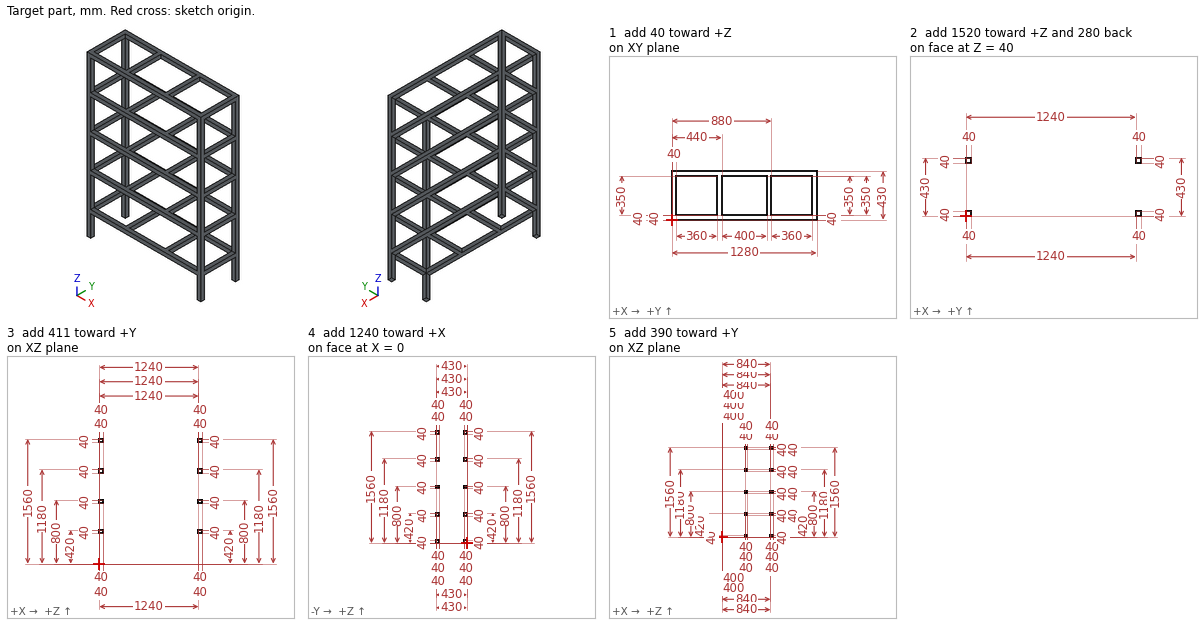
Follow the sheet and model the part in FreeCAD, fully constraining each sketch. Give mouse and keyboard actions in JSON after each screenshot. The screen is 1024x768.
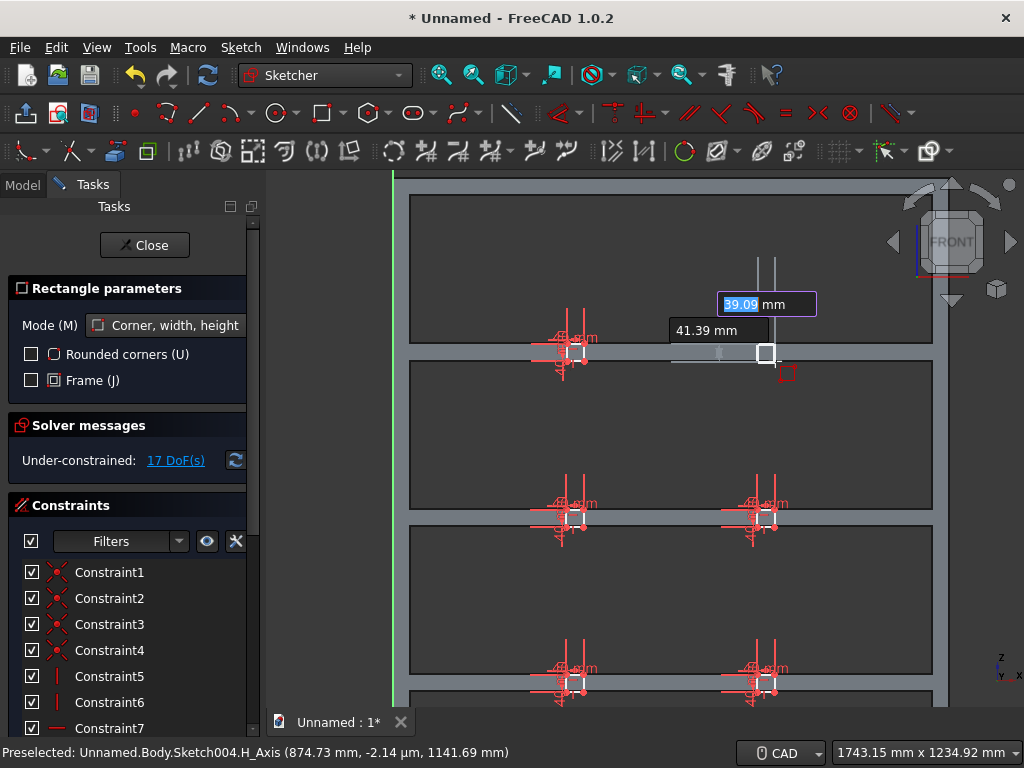
{"action": "type", "text": "40"}
{"action": "key", "text": "Tab"}
{"action": "type", "text": "40"}
{"action": "key", "text": "Return"}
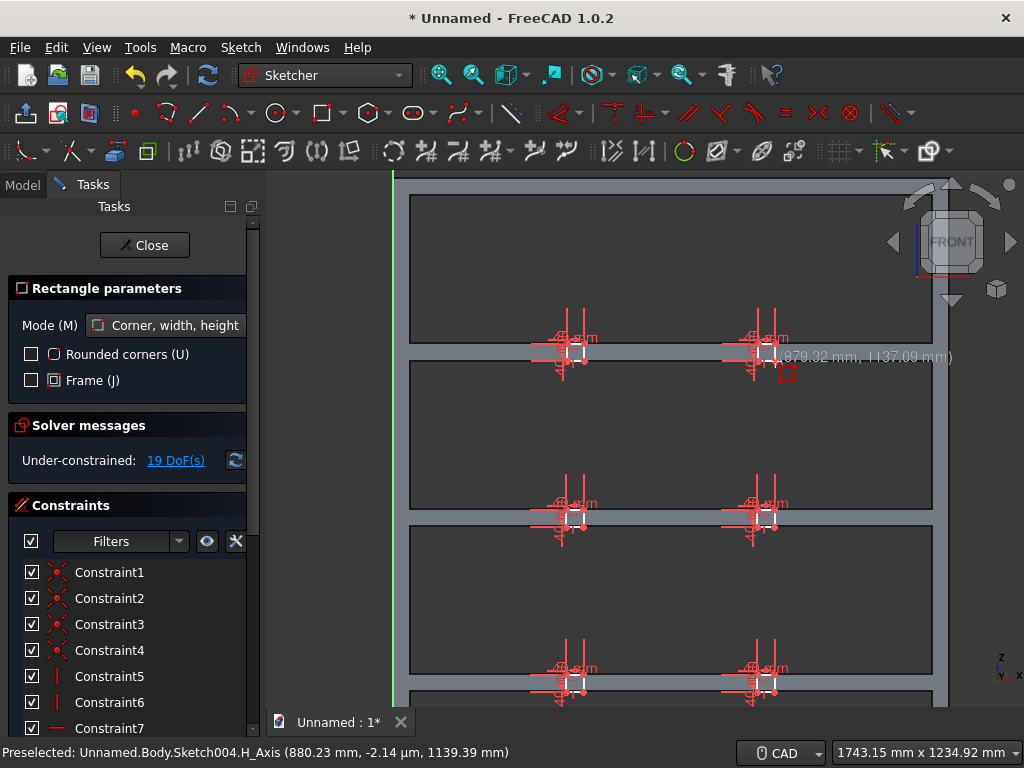
{"action": "scroll", "coordinate": [567, 343], "scroll_direction": "down", "scroll_amount": 3}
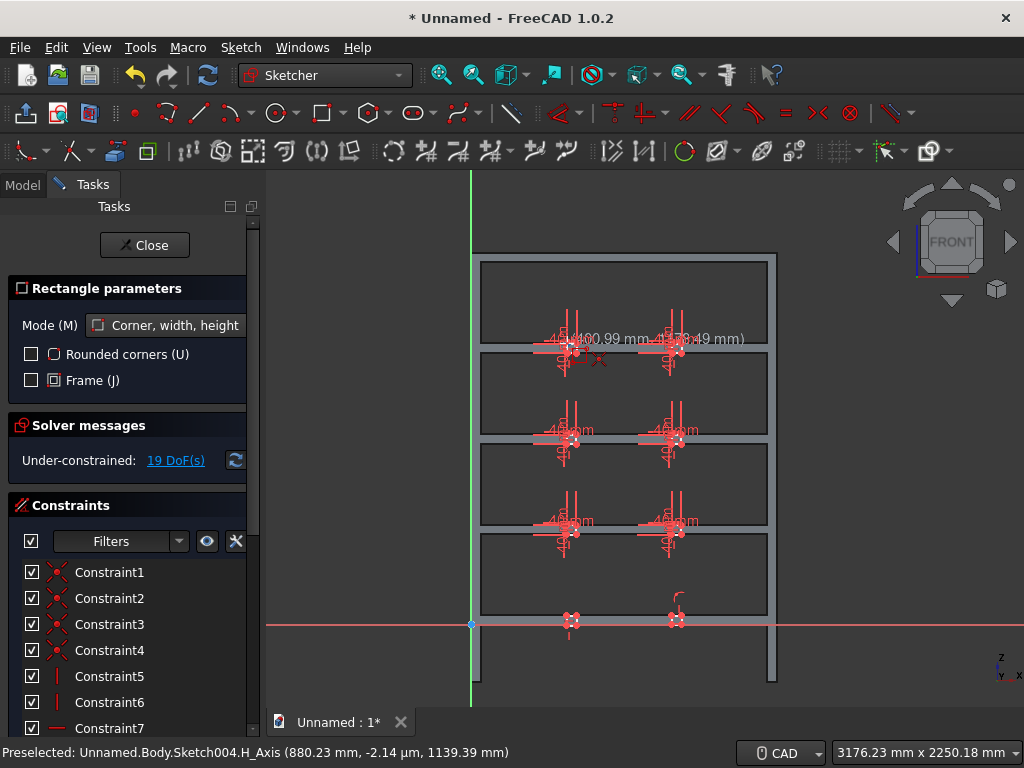
{"action": "scroll", "coordinate": [672, 253], "scroll_direction": "up", "scroll_amount": 3}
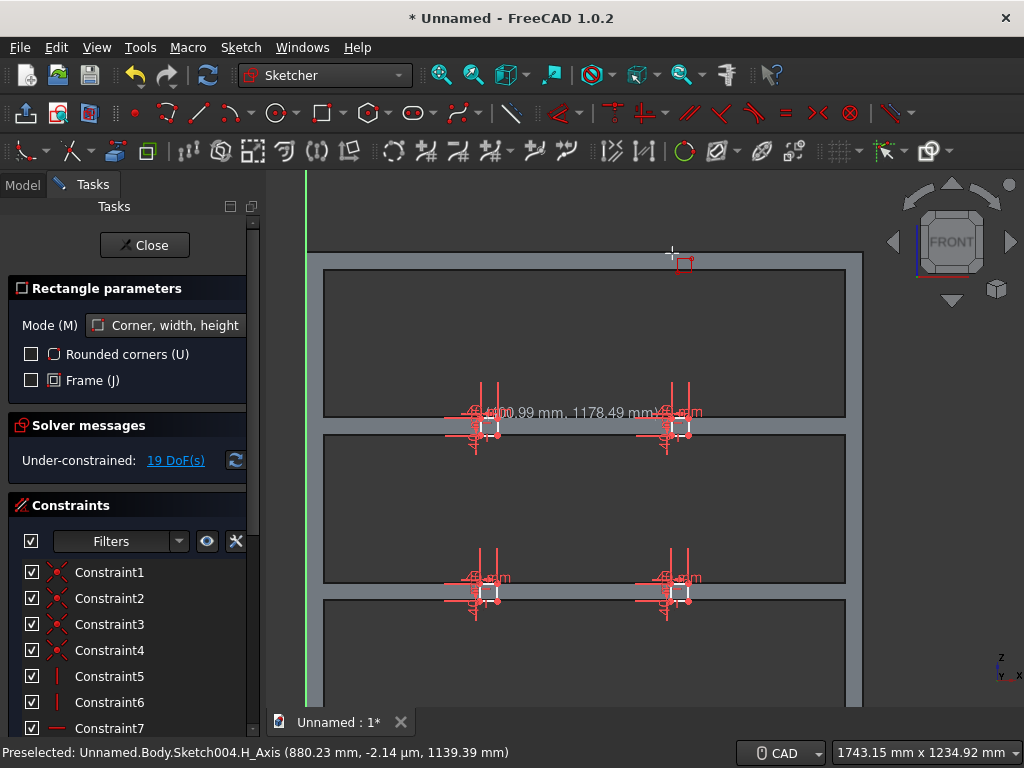
{"action": "left_click", "coordinate": [671, 252]}
{"action": "mouse_move", "coordinate": [689, 270]}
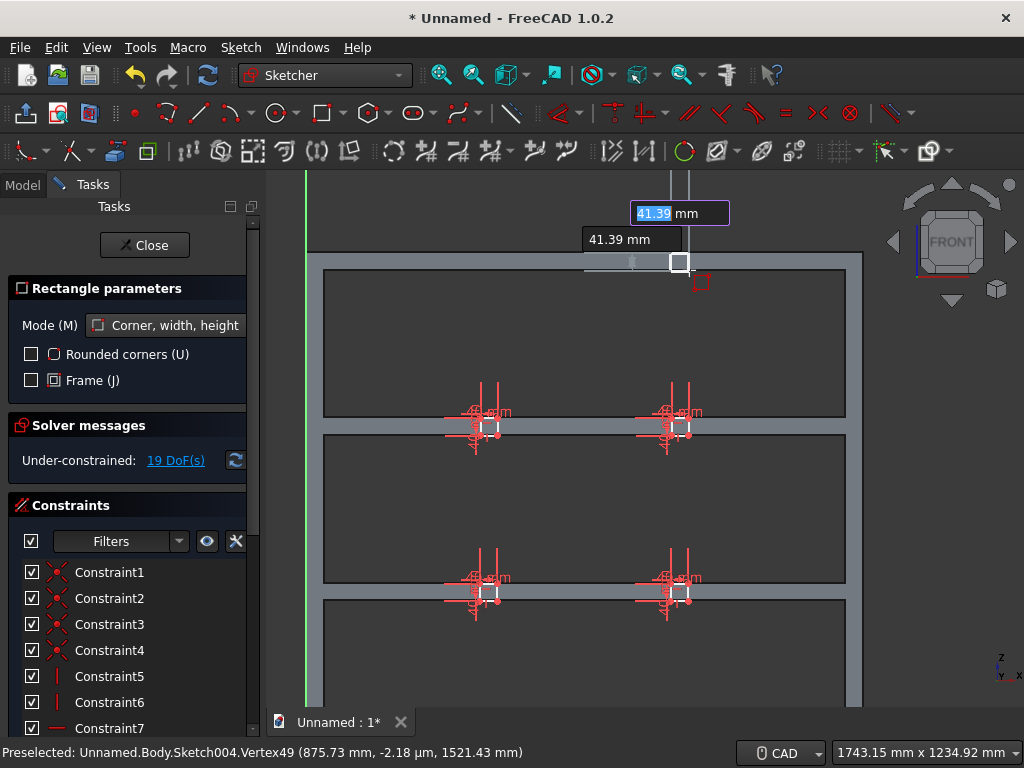
{"action": "type", "text": "40"}
{"action": "key", "text": "Tab"}
{"action": "type", "text": "40"}
{"action": "key", "text": "Return"}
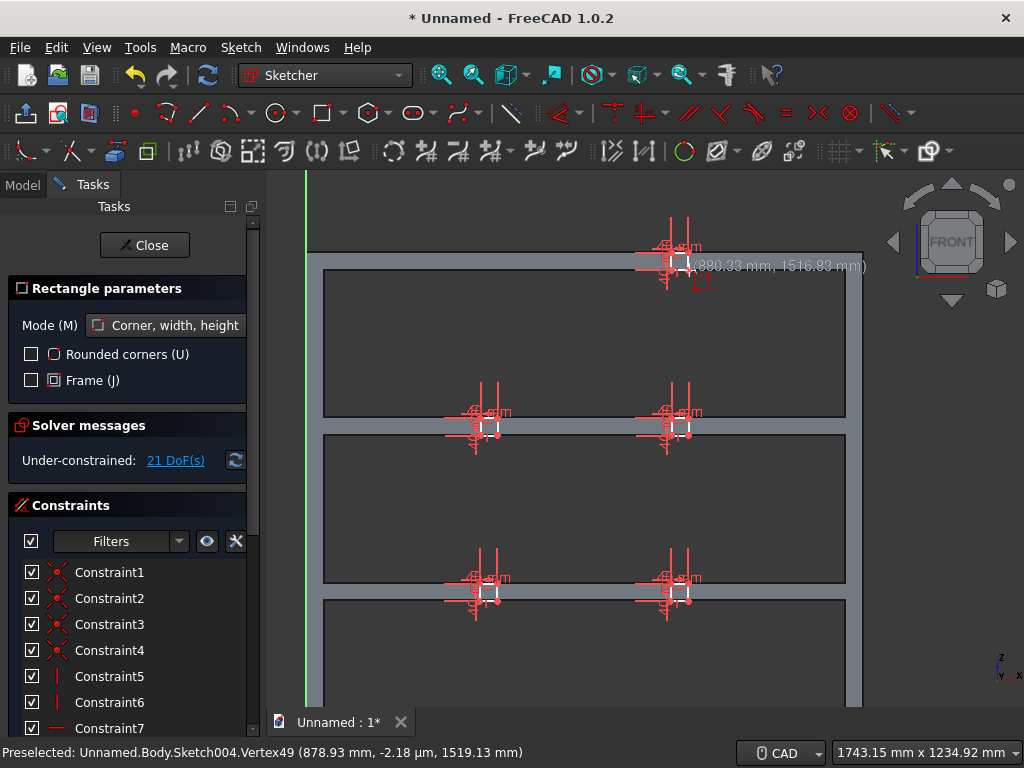
{"action": "left_click", "coordinate": [480, 252]}
{"action": "mouse_move", "coordinate": [498, 270]}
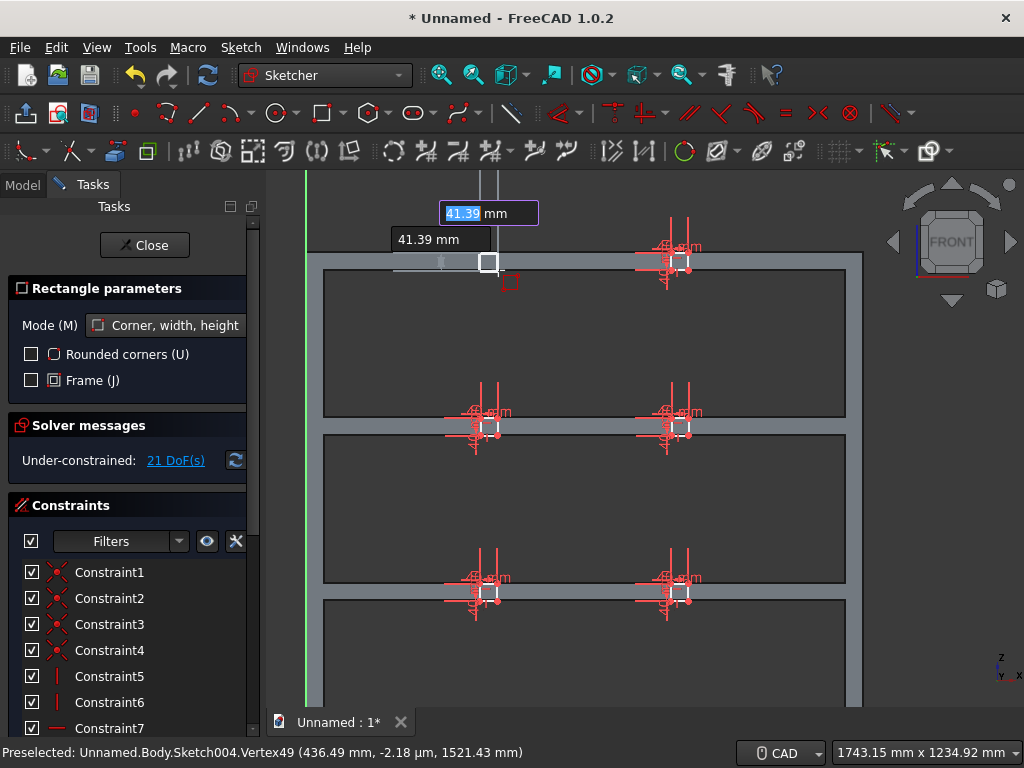
{"action": "type", "text": "40"}
{"action": "key", "text": "Tab"}
{"action": "type", "text": "40"}
{"action": "key", "text": "Return"}
{"action": "key", "text": "Escape"}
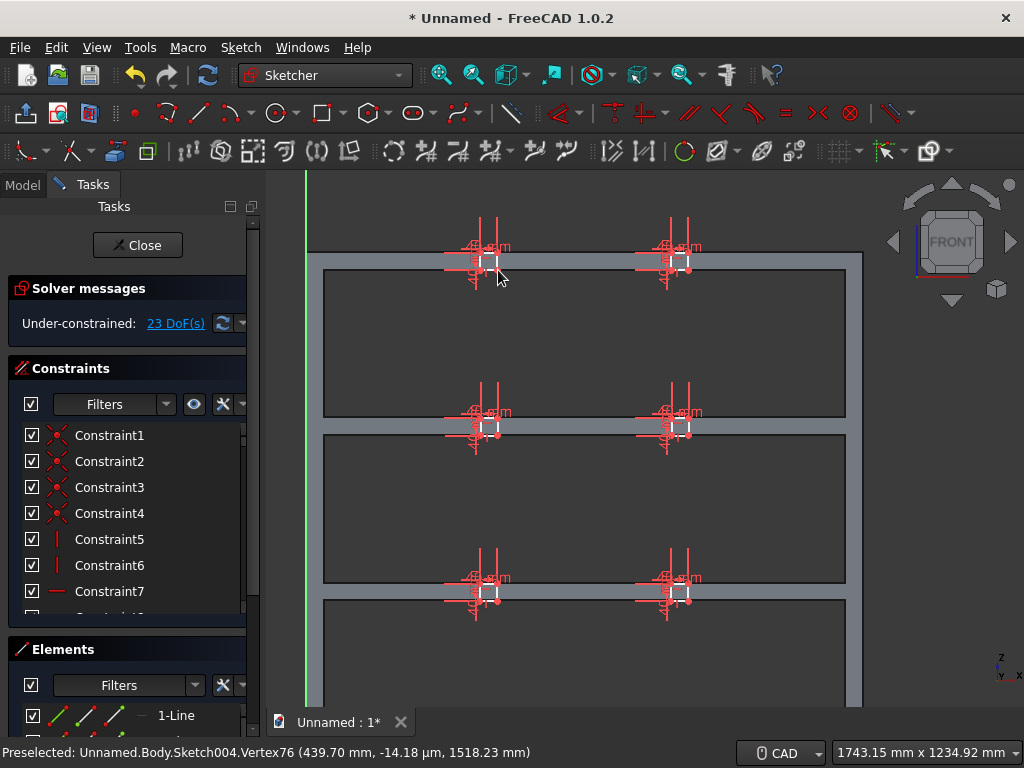
{"action": "scroll", "coordinate": [673, 253], "scroll_direction": "down", "scroll_amount": 3}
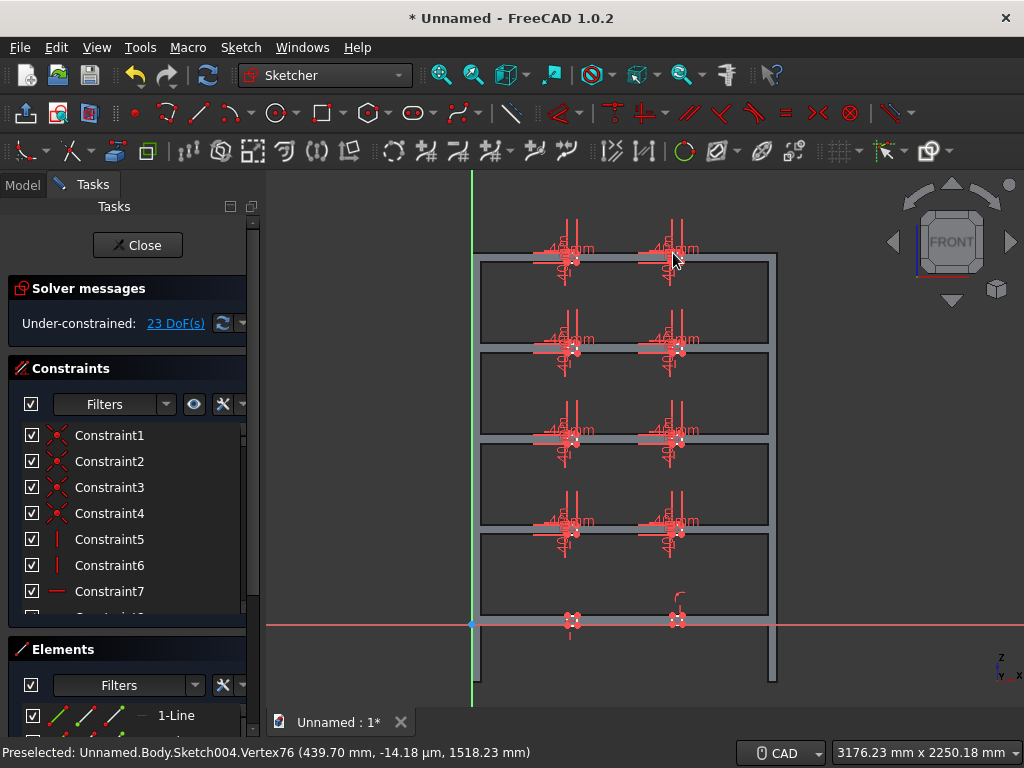
{"action": "scroll", "coordinate": [567, 626], "scroll_direction": "up", "scroll_amount": 2}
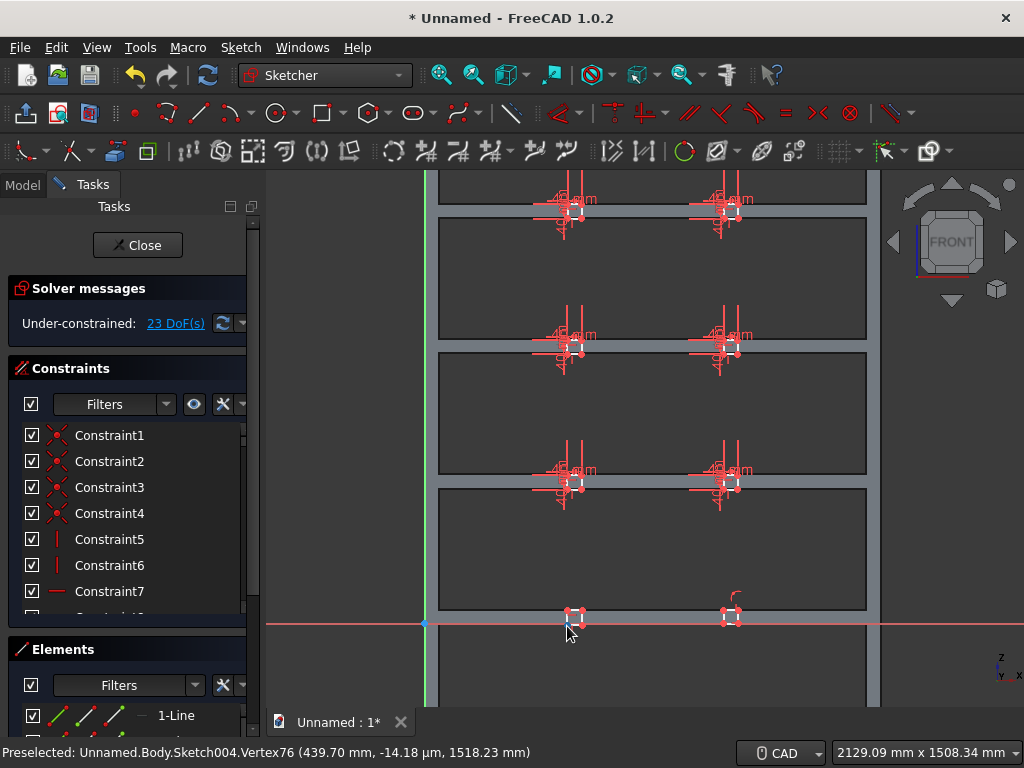
{"action": "left_click", "coordinate": [567, 625]}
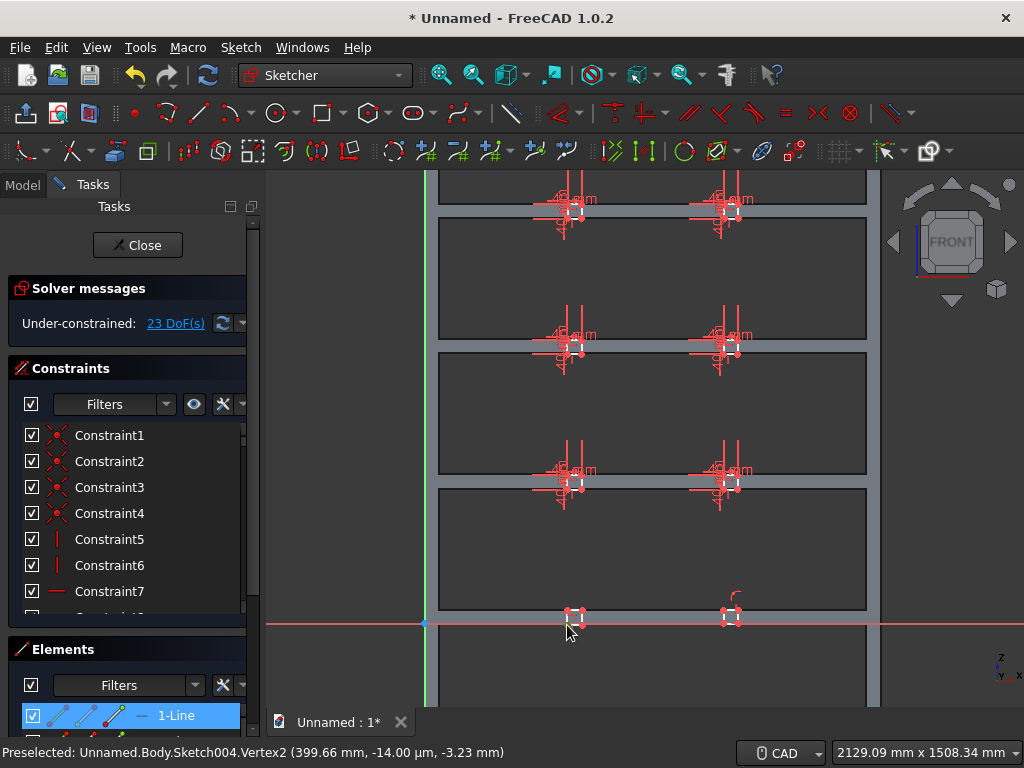
{"action": "left_click", "coordinate": [334, 624]}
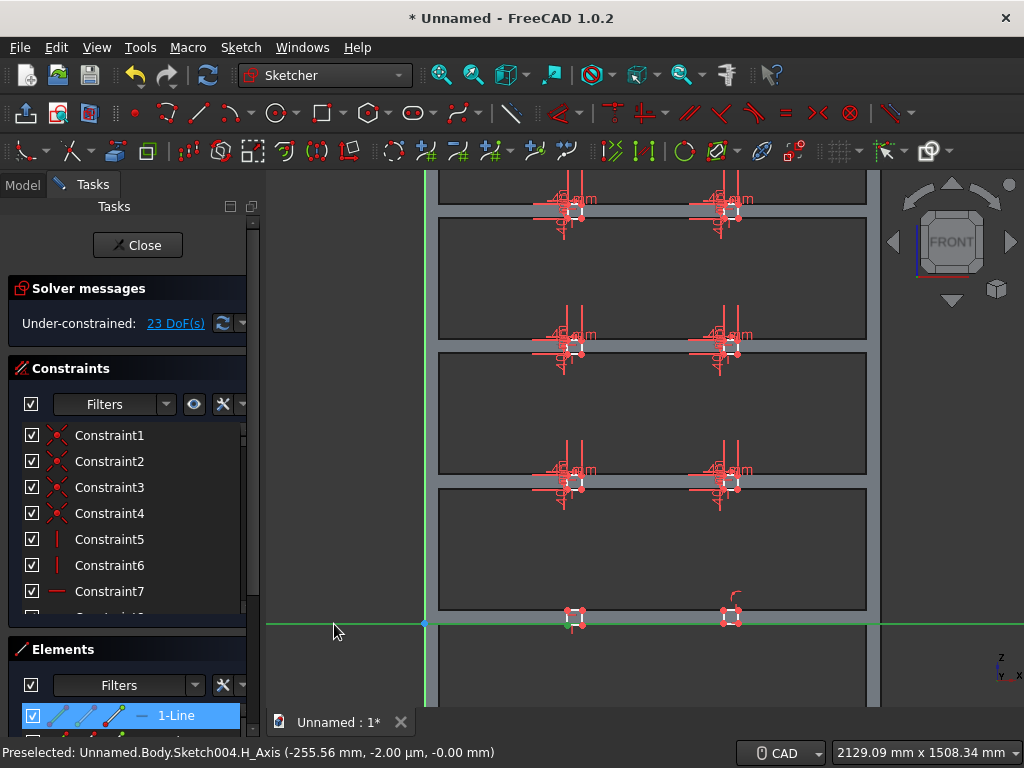
{"action": "left_click", "coordinate": [614, 114]}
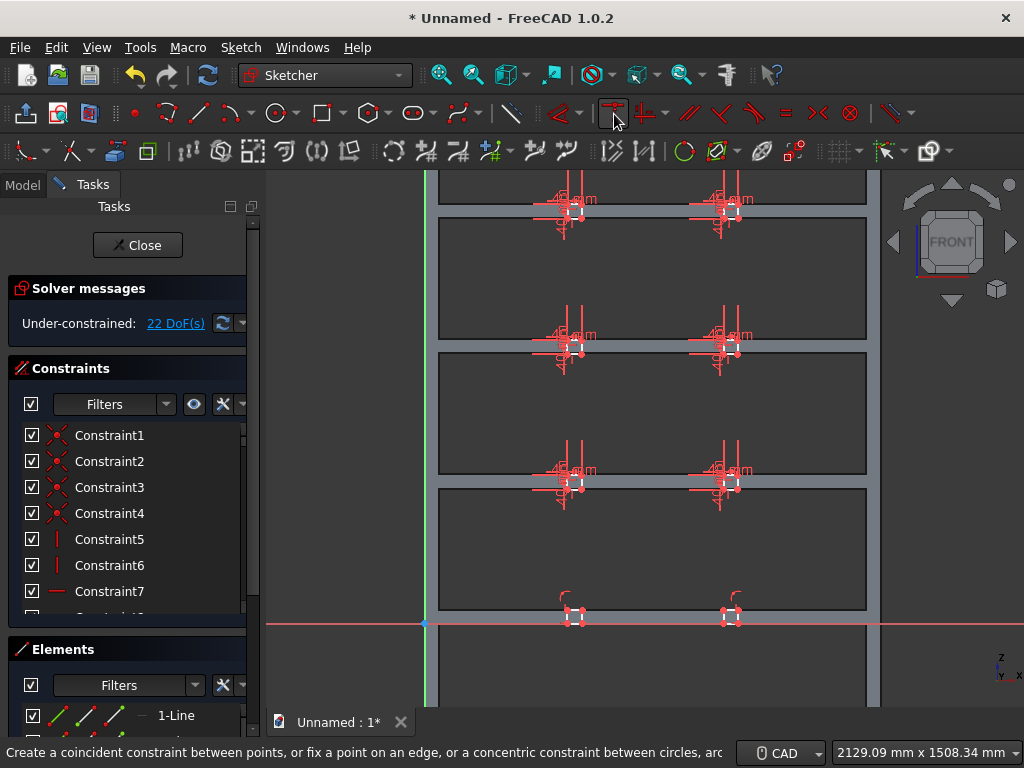
{"action": "left_click", "coordinate": [558, 114]}